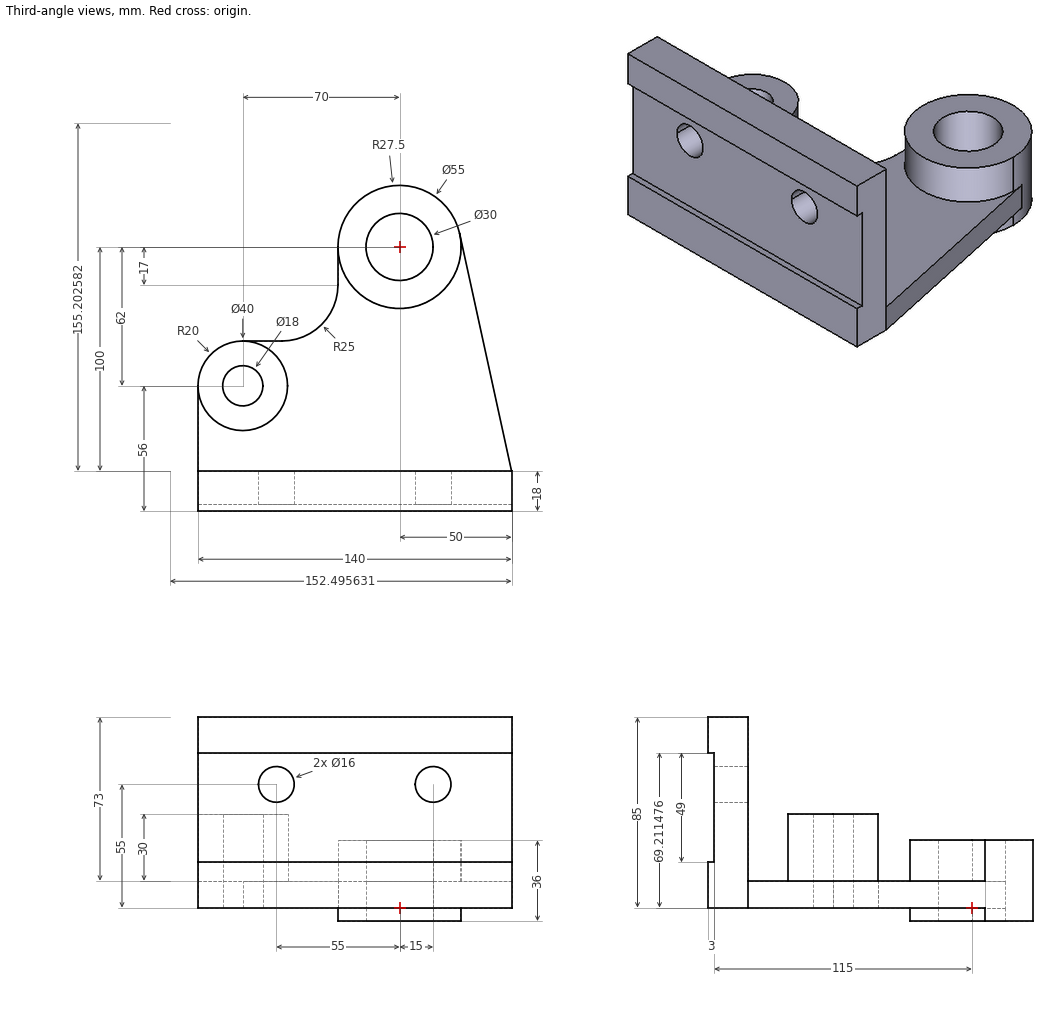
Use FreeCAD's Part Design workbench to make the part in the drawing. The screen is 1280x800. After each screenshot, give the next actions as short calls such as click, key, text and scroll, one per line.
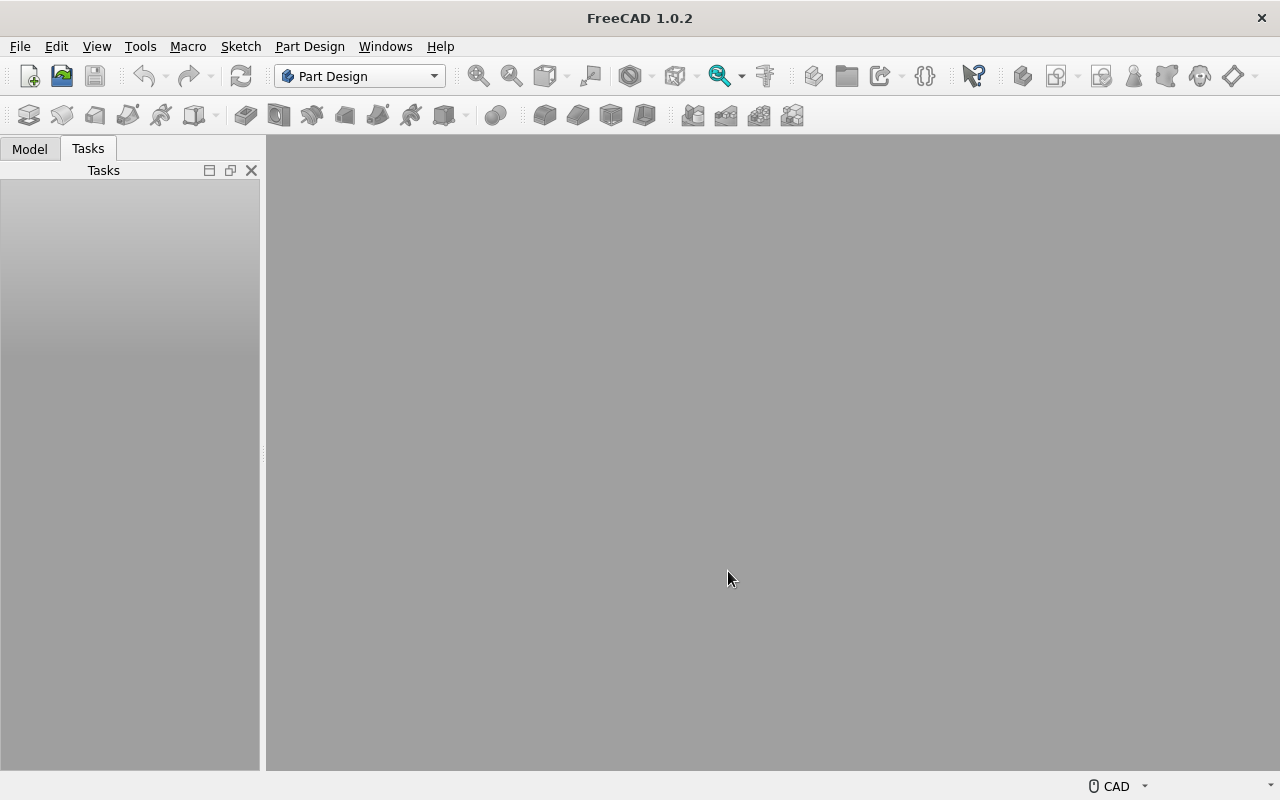
click(29, 76)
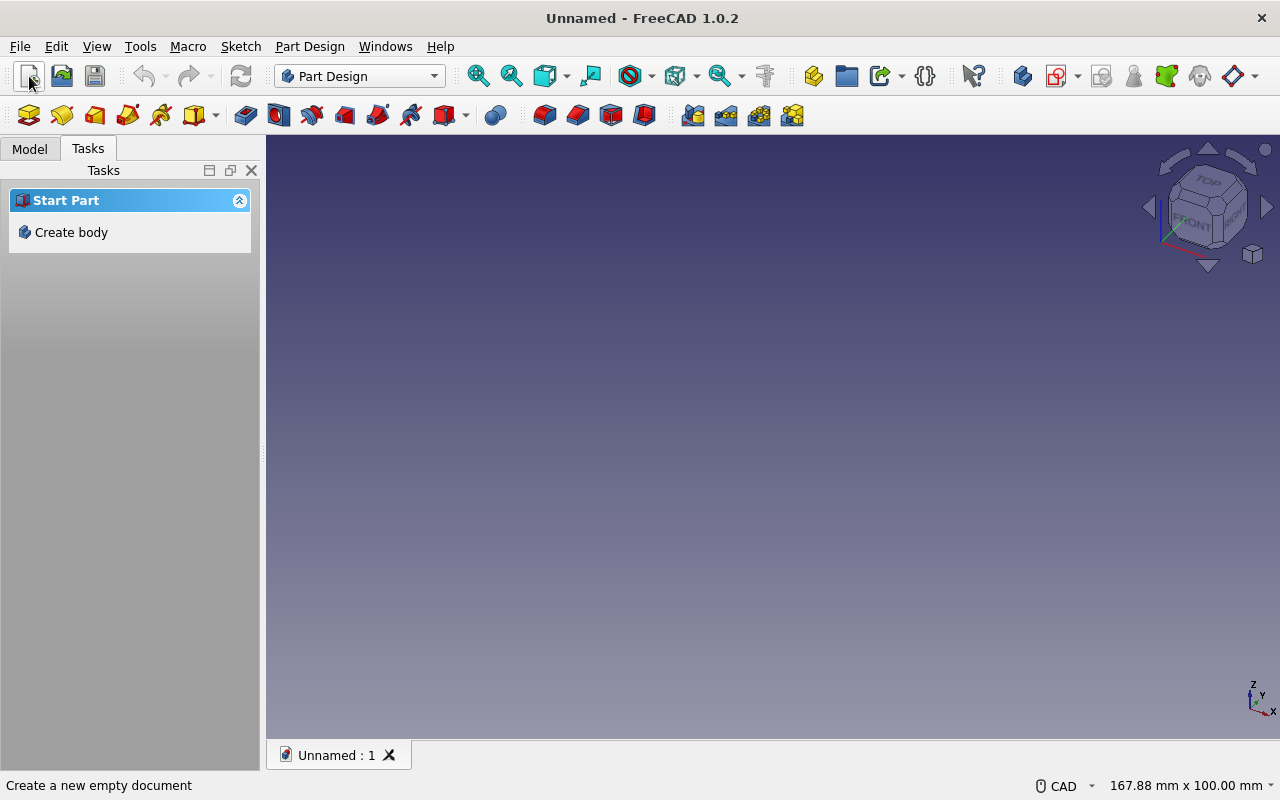
click(1056, 76)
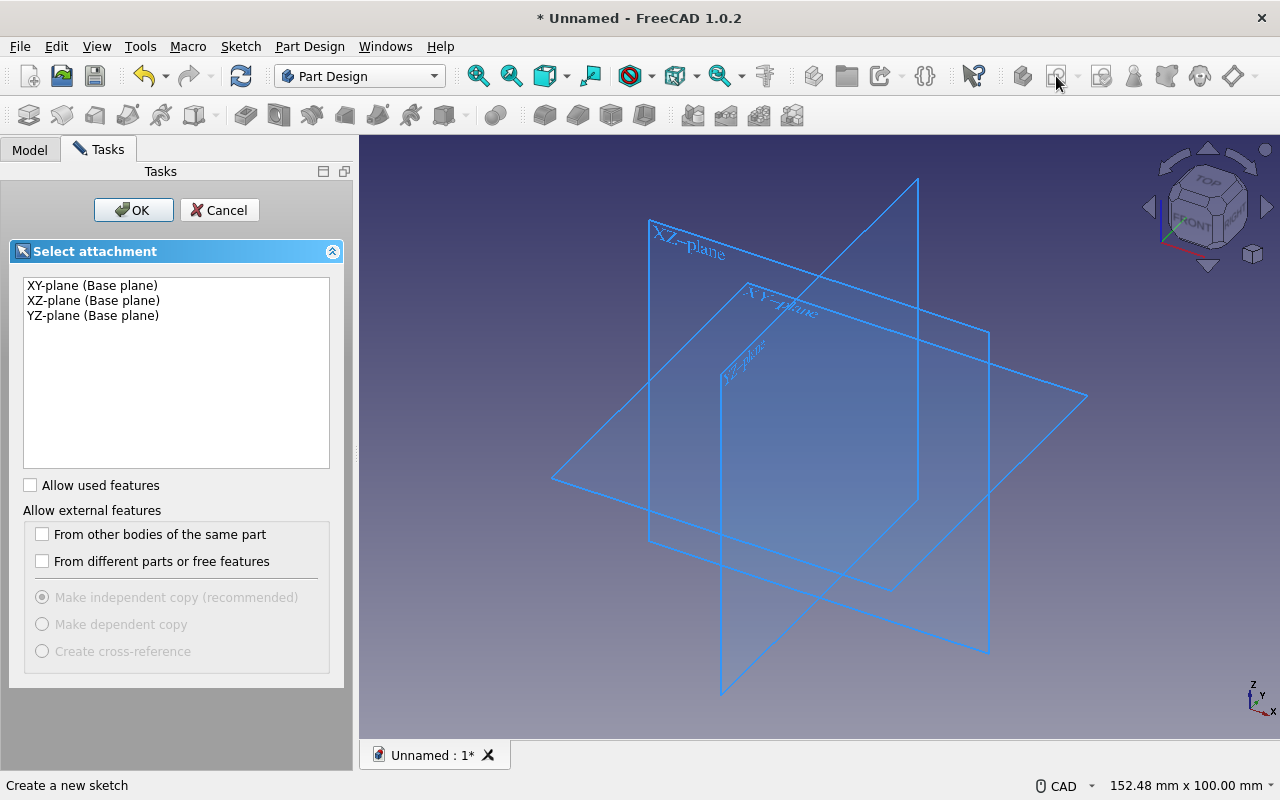
click(84, 286)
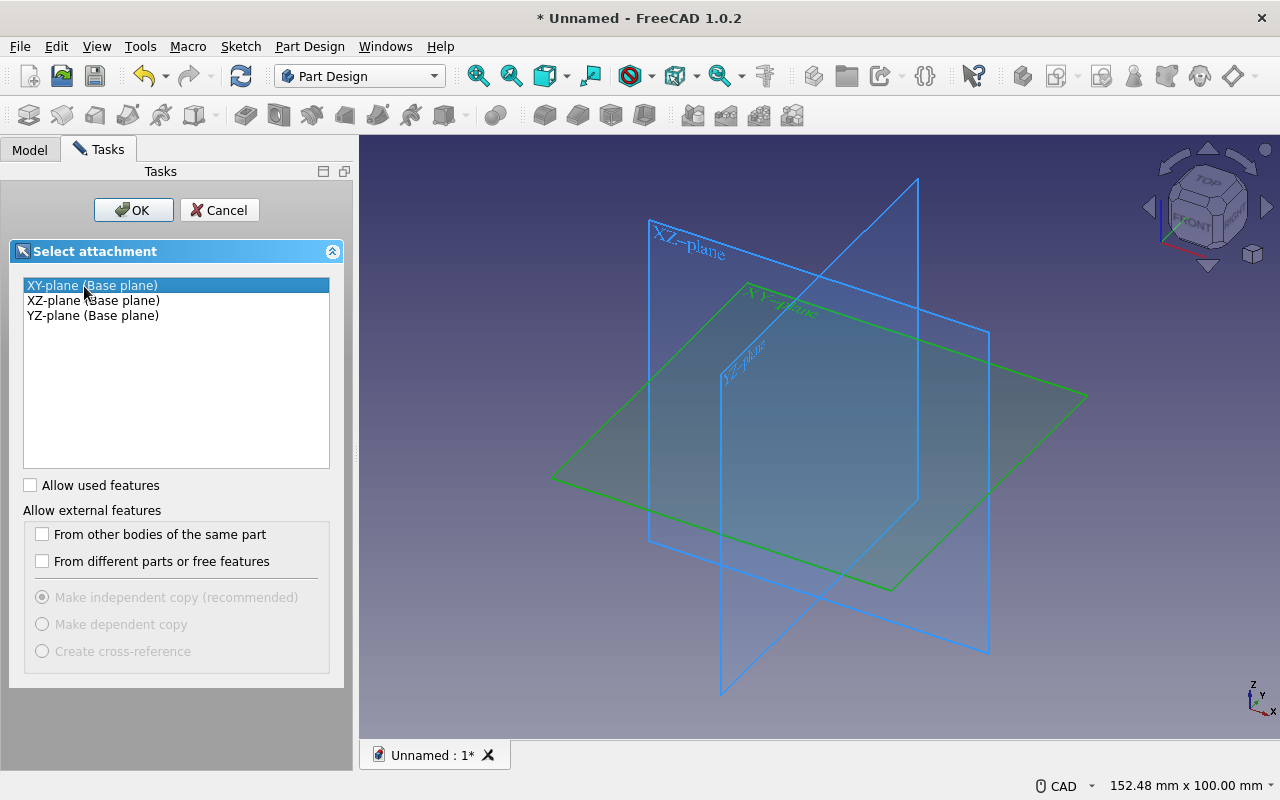
click(134, 210)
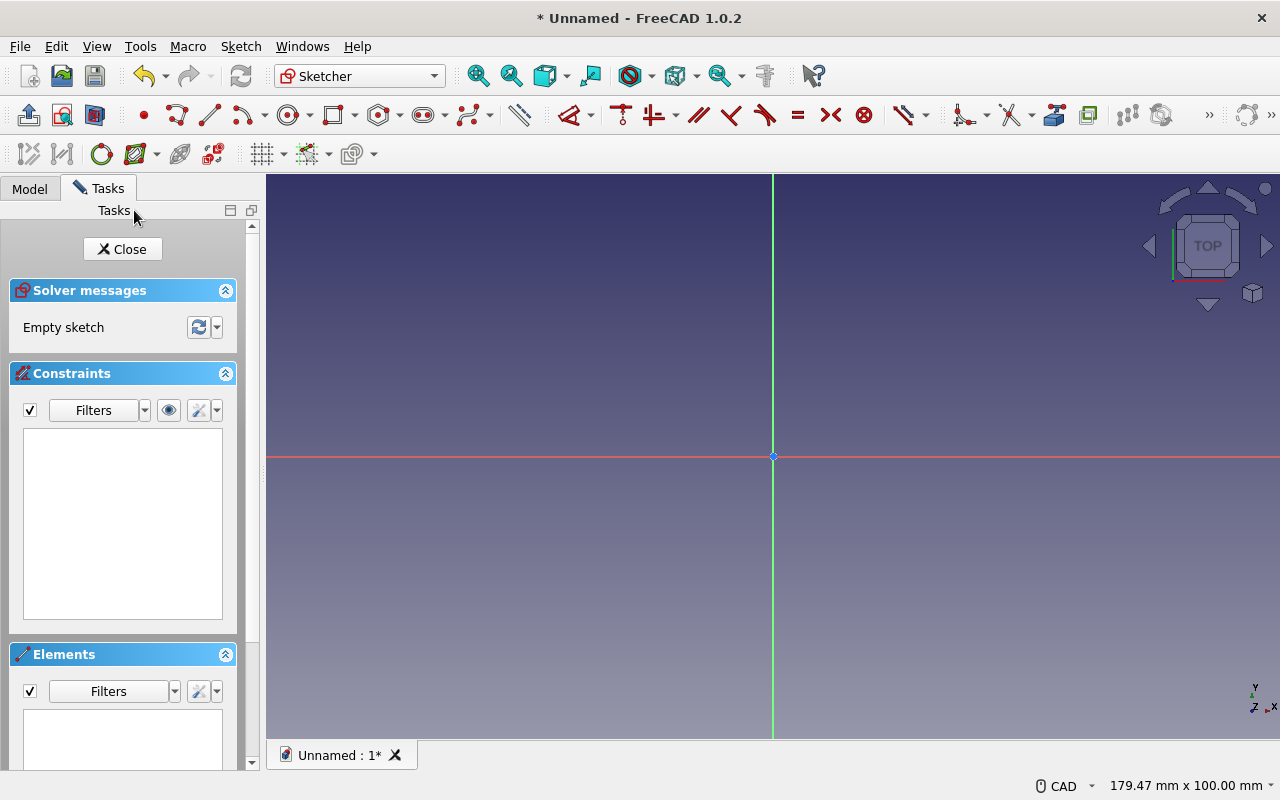
scroll(741, 248, down, 4)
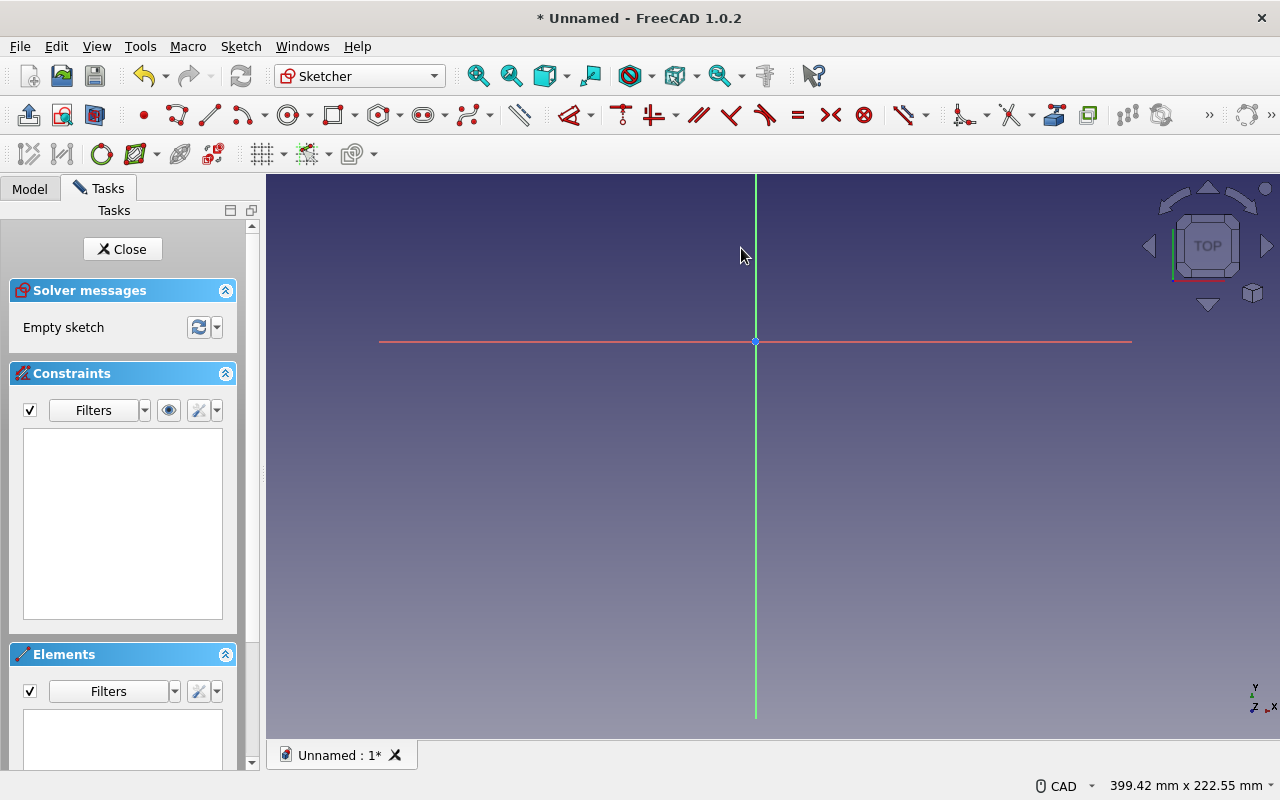
click(177, 116)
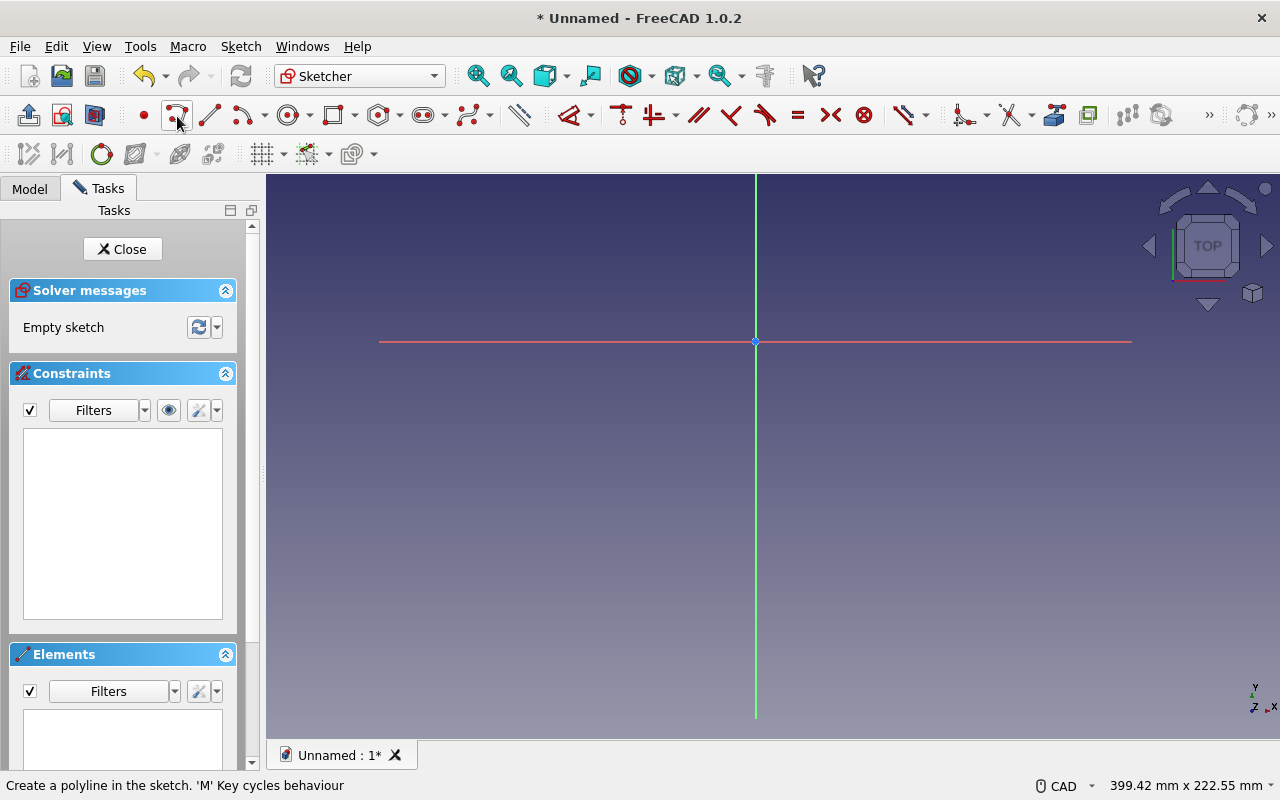
click(527, 499)
click(527, 641)
click(883, 641)
click(883, 596)
click(824, 327)
right_click(824, 327)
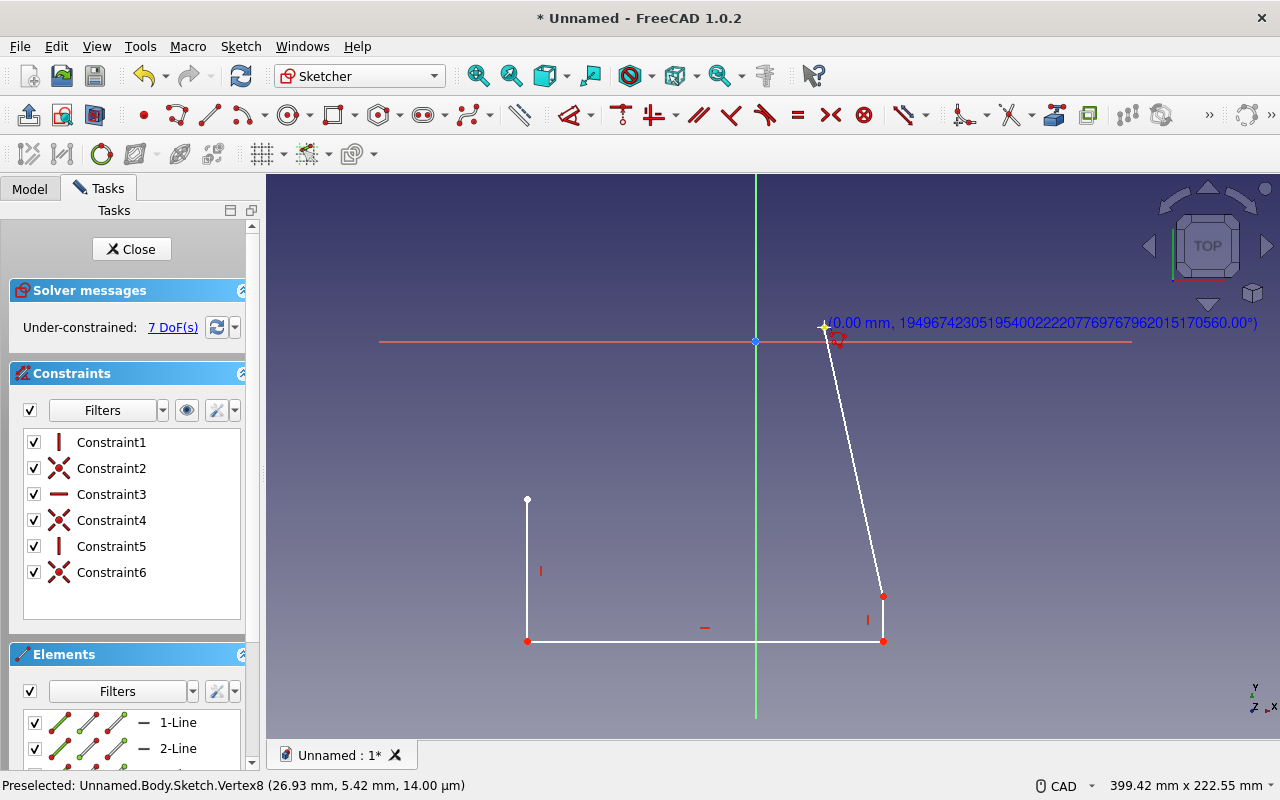
key(g)
key(l)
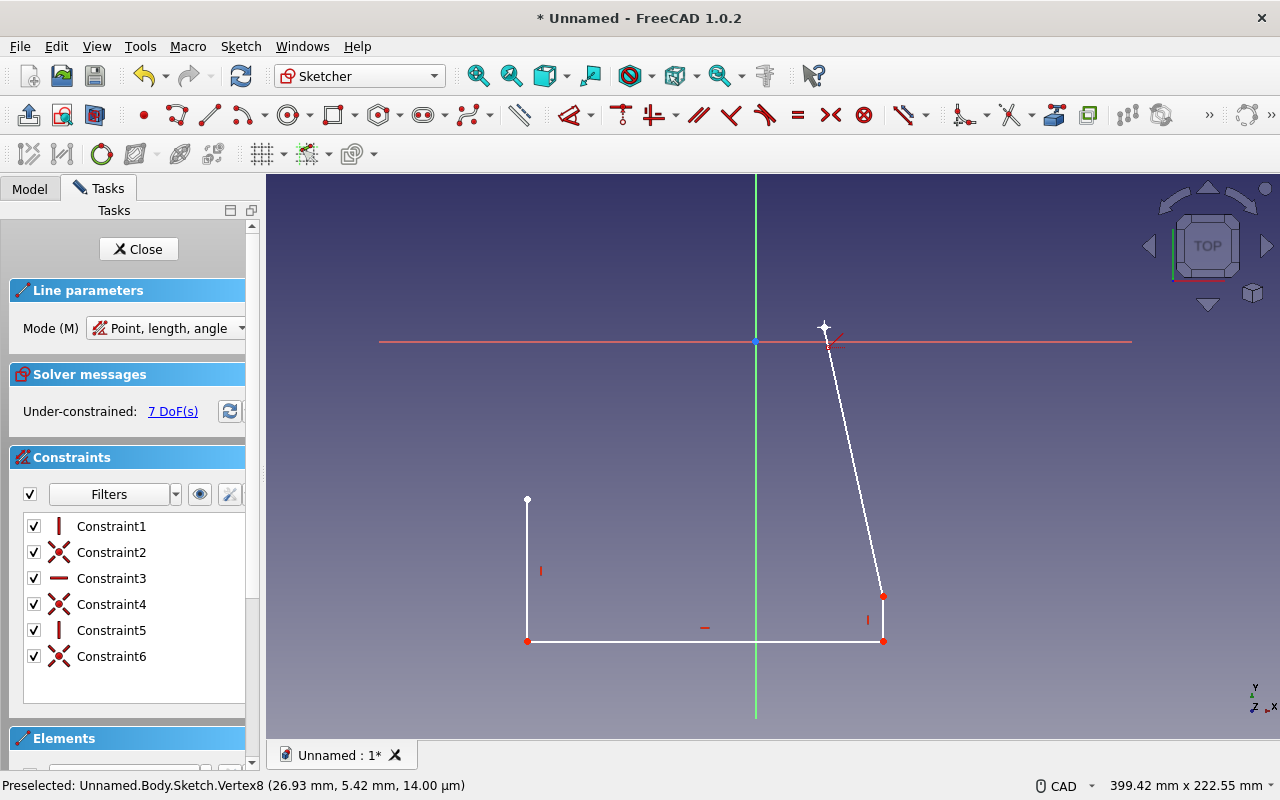
click(686, 342)
click(686, 385)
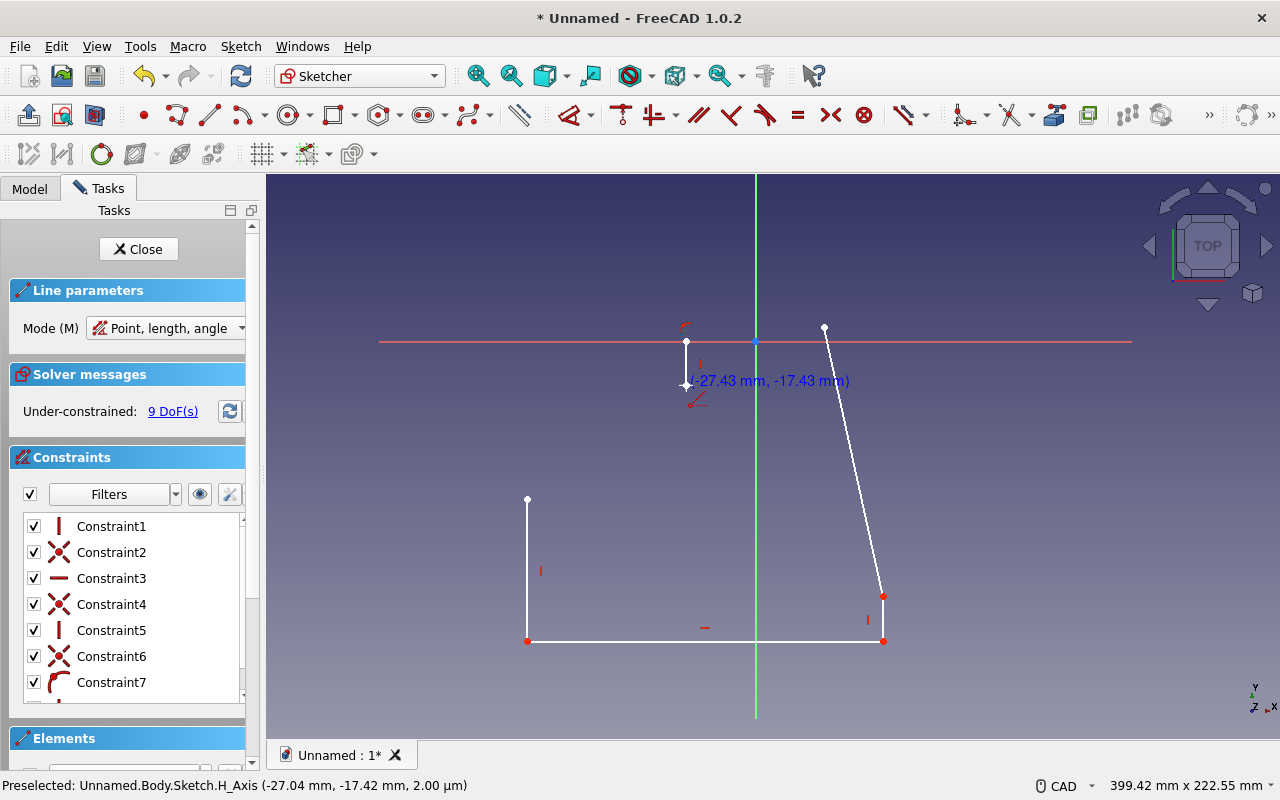
click(622, 448)
click(578, 448)